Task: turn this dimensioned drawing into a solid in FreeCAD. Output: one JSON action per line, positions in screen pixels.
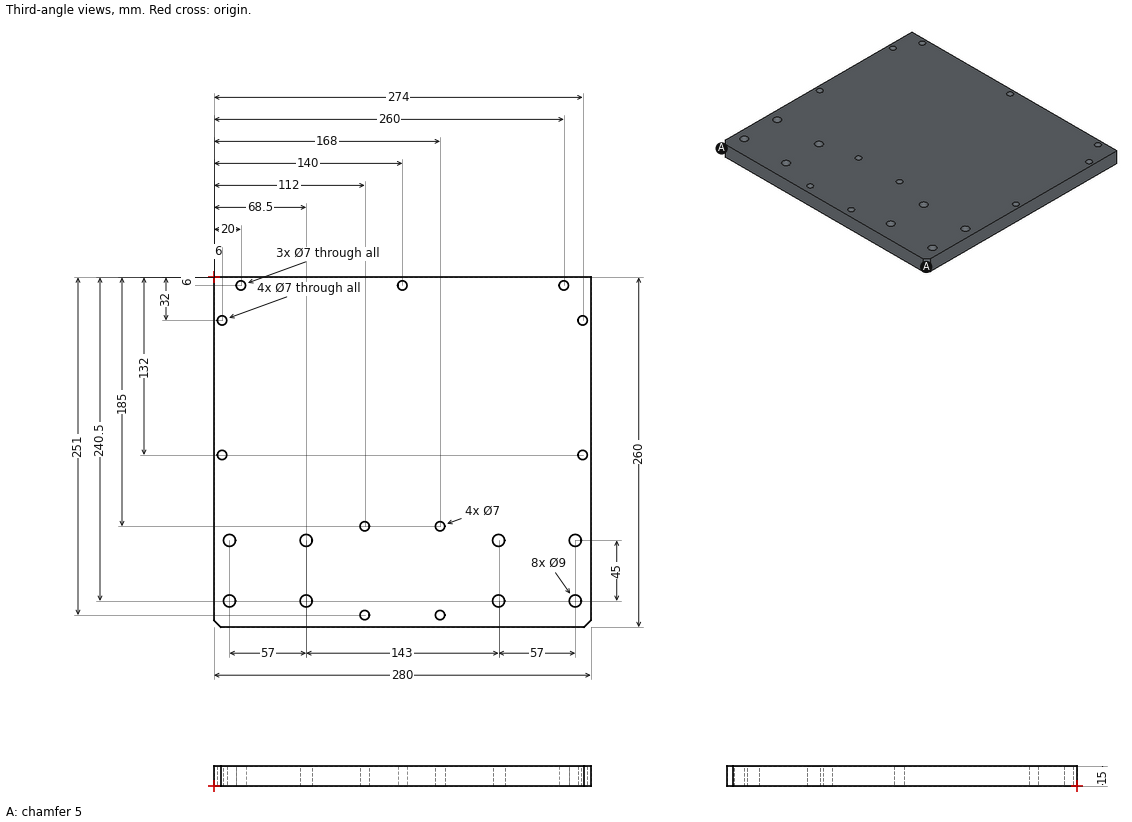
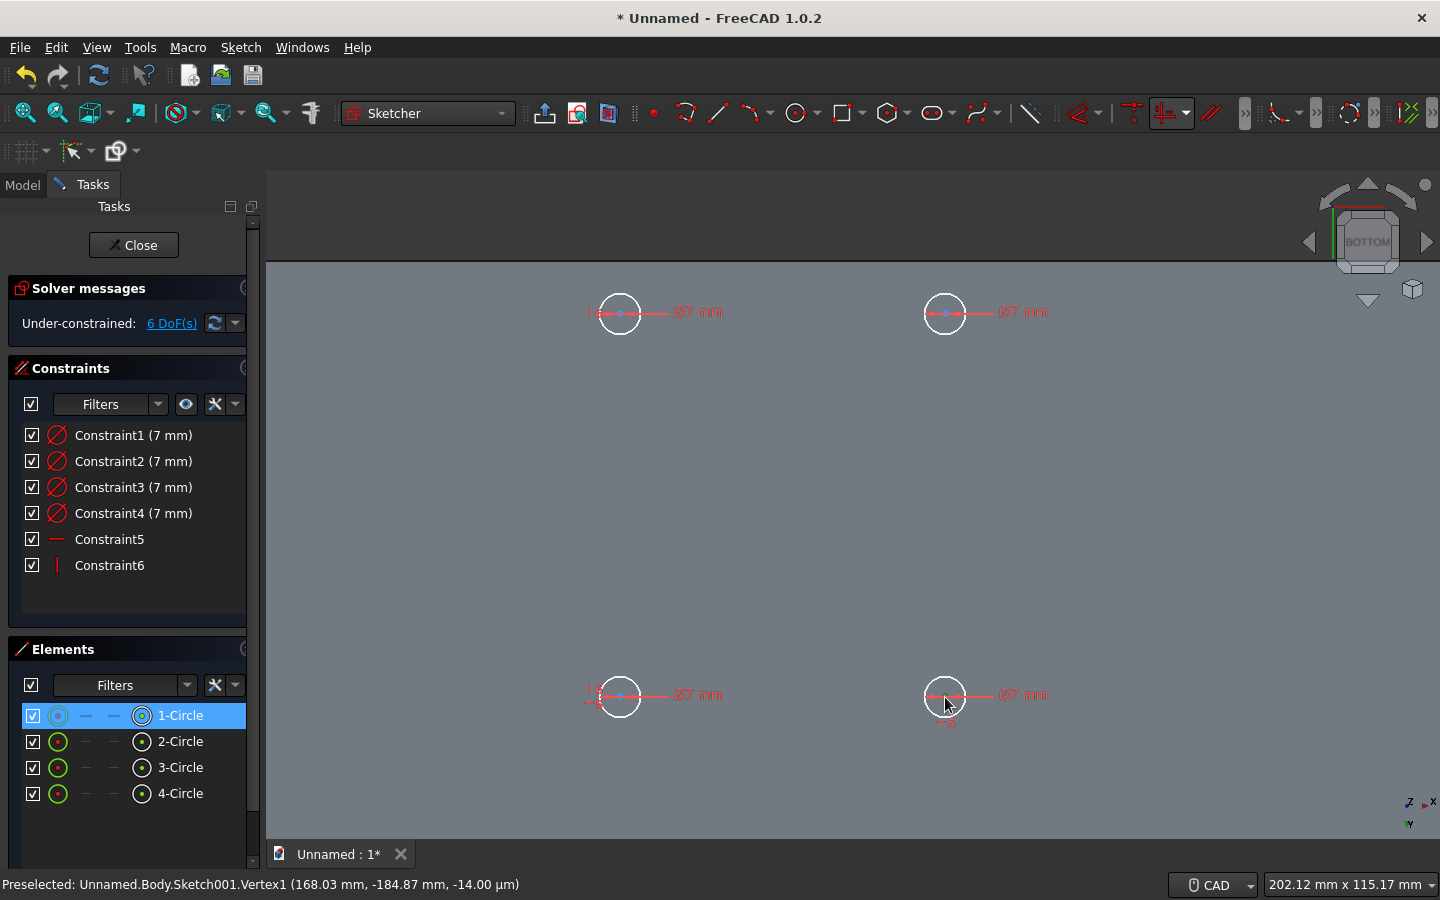
{"action": "left_click", "coordinate": [945, 314]}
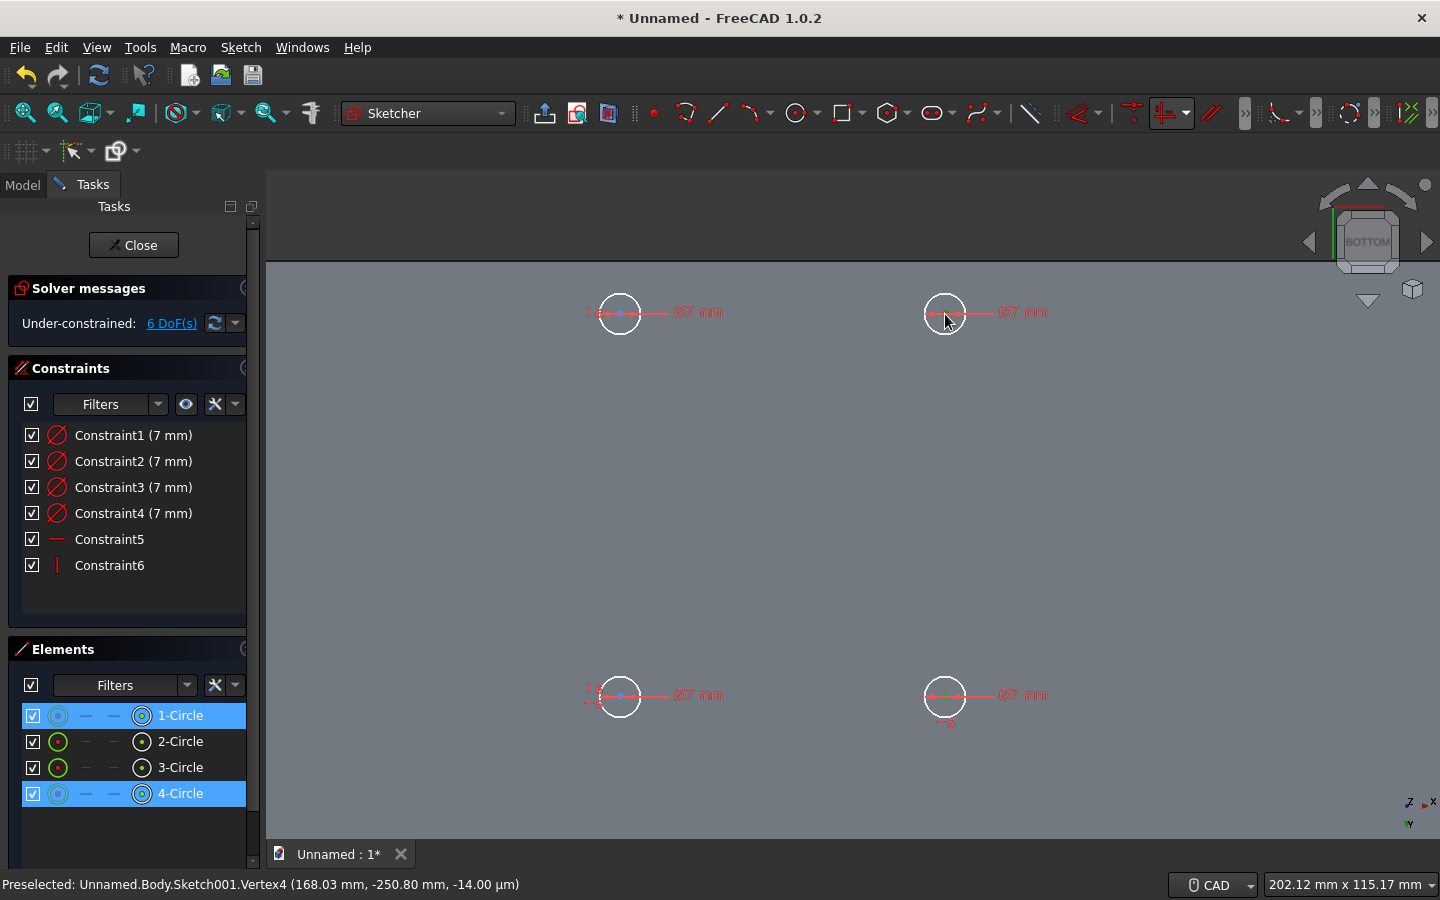
{"action": "left_click", "coordinate": [1188, 114]}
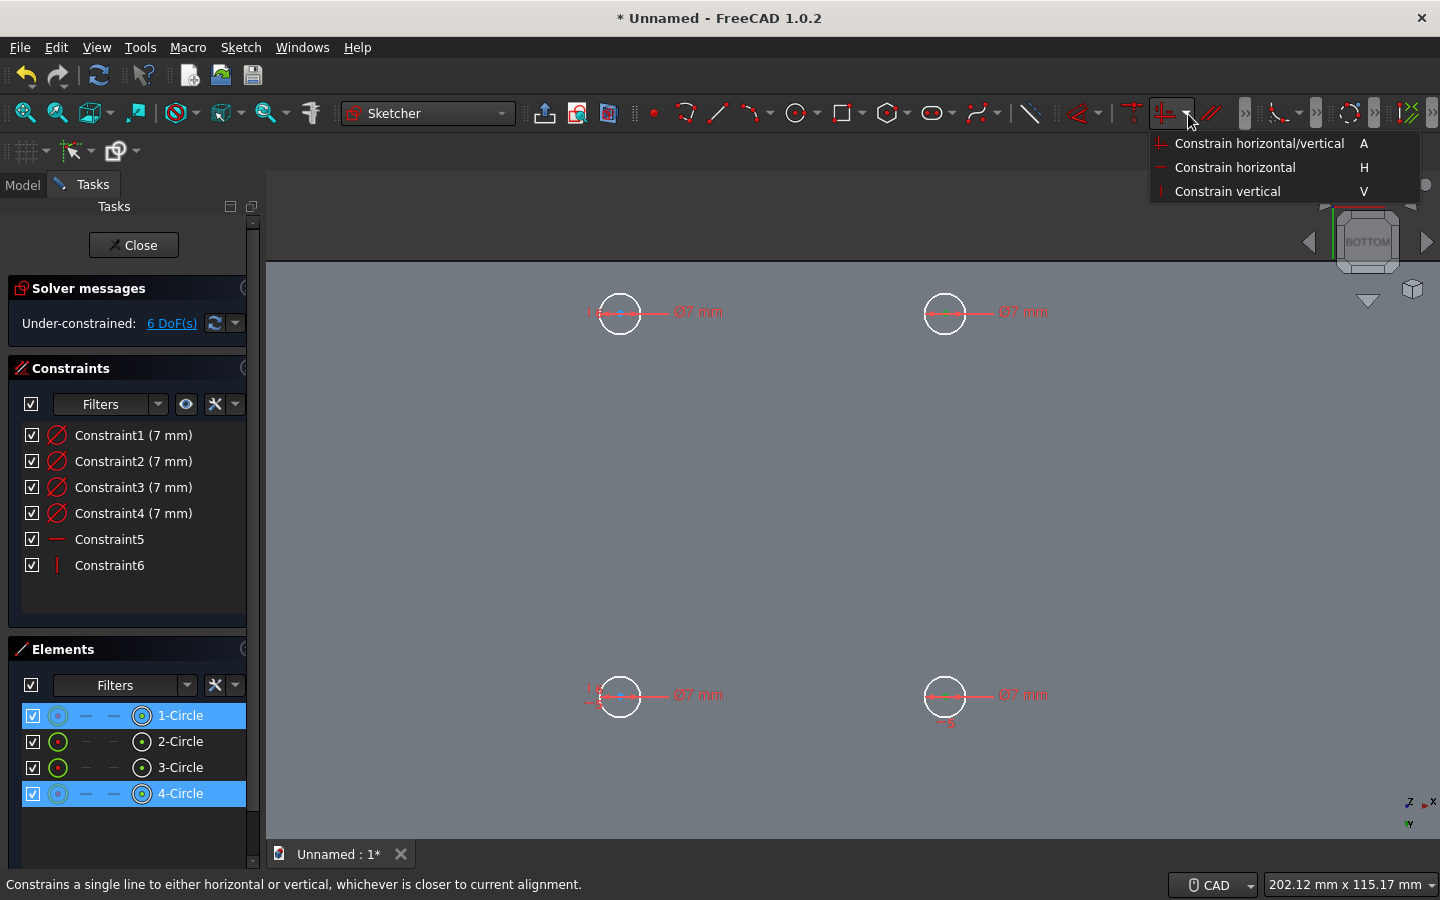
{"action": "left_click", "coordinate": [1285, 191]}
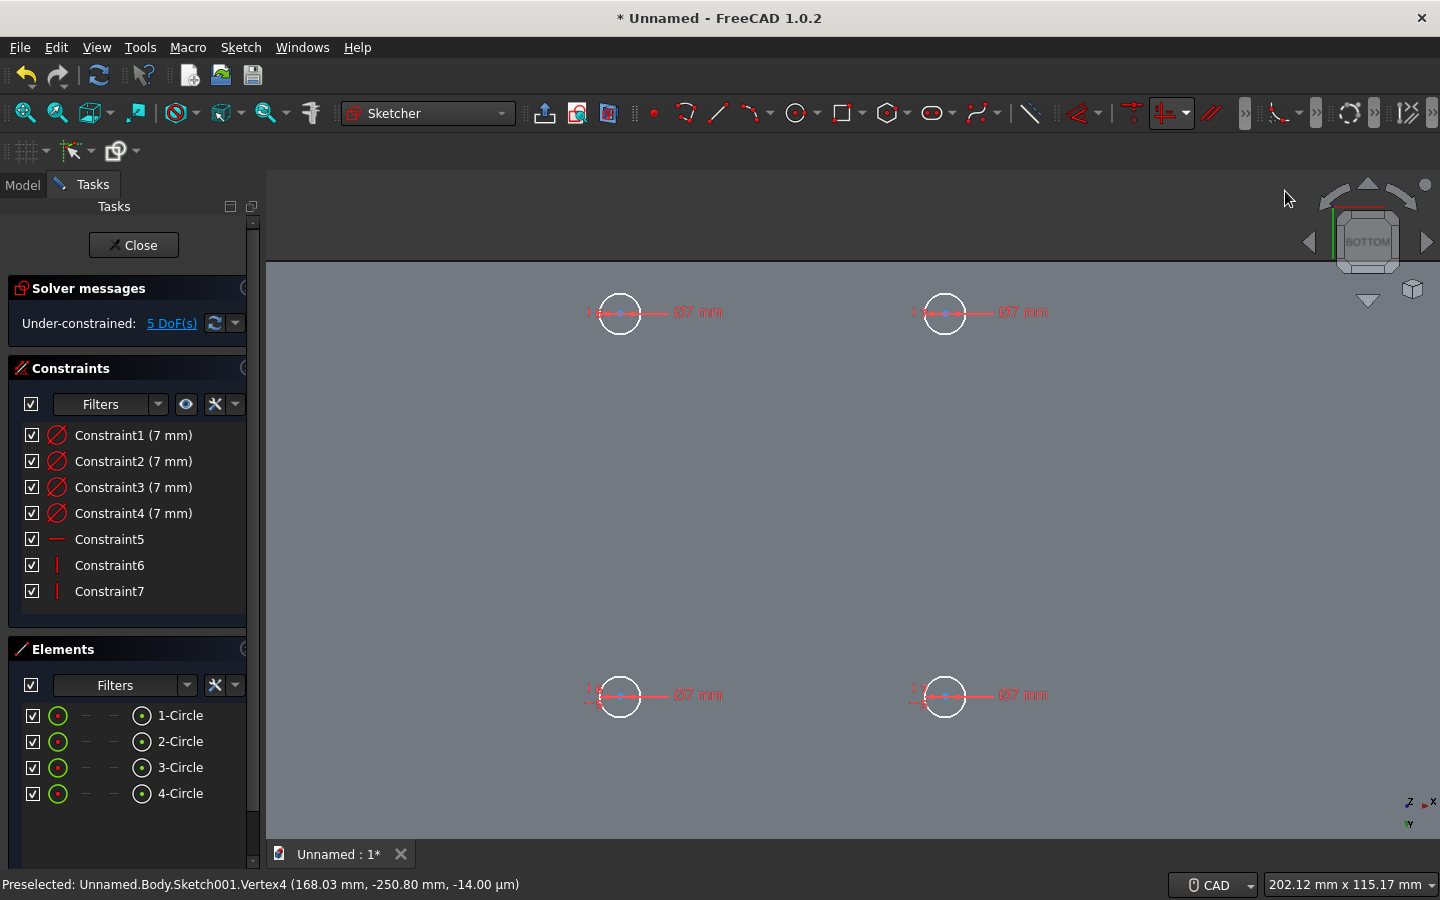
{"action": "left_click", "coordinate": [620, 314]}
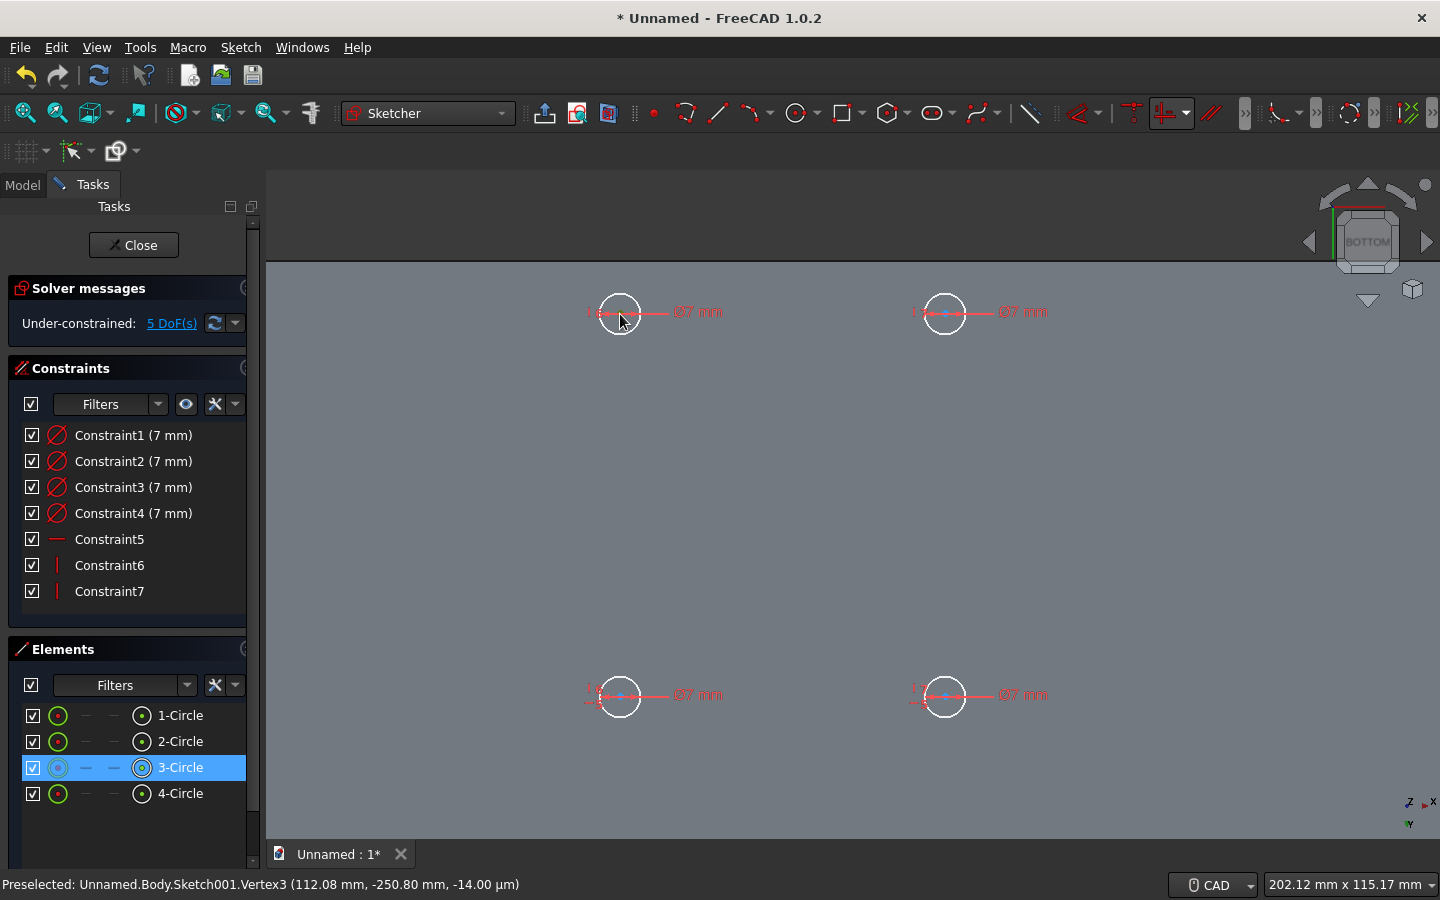
{"action": "left_click", "coordinate": [945, 314]}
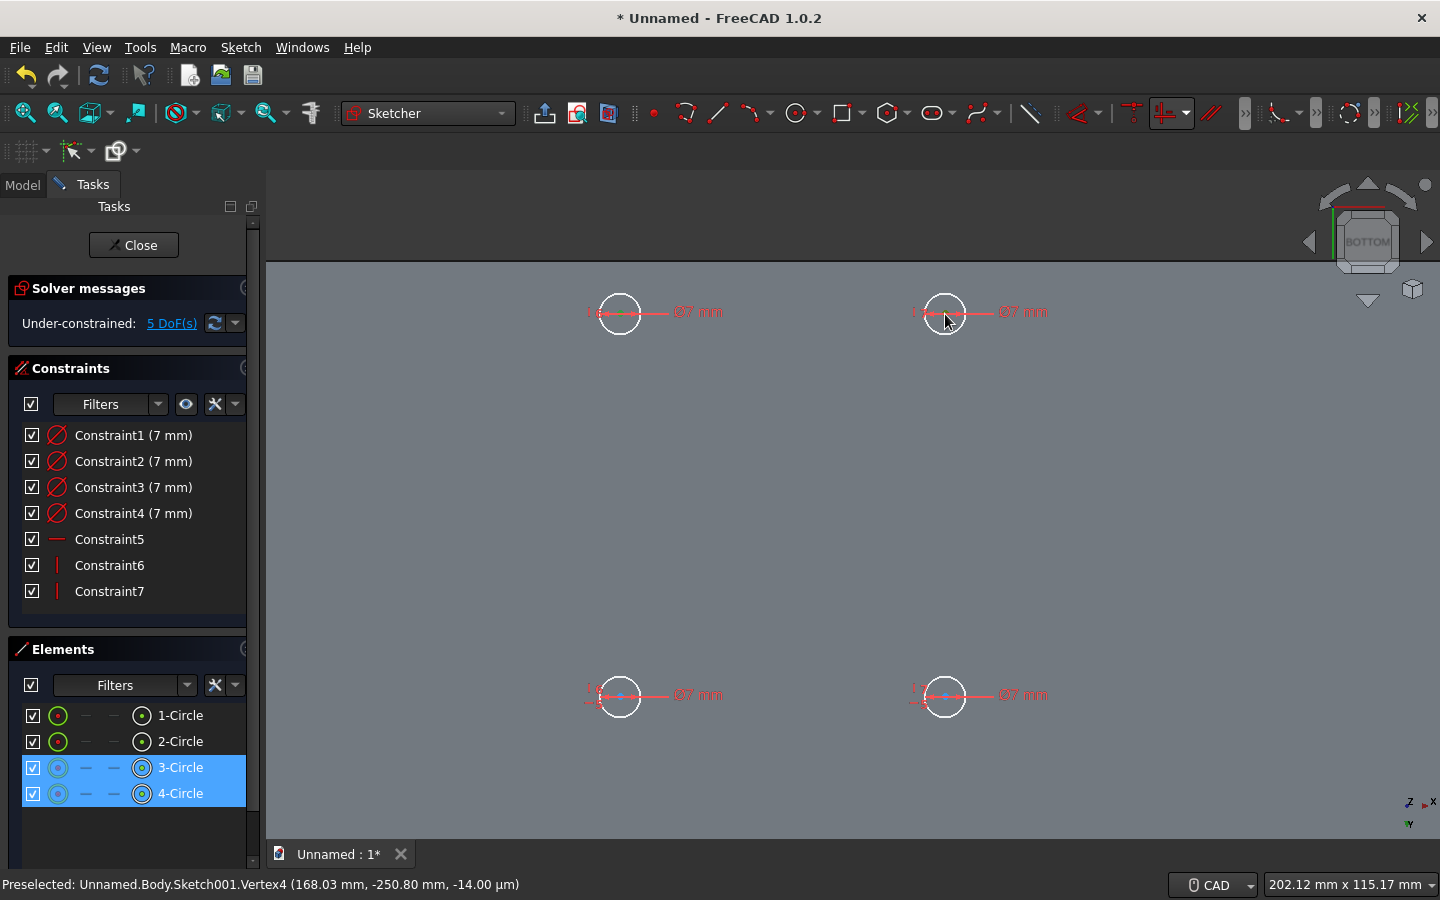
{"action": "key", "text": "h"}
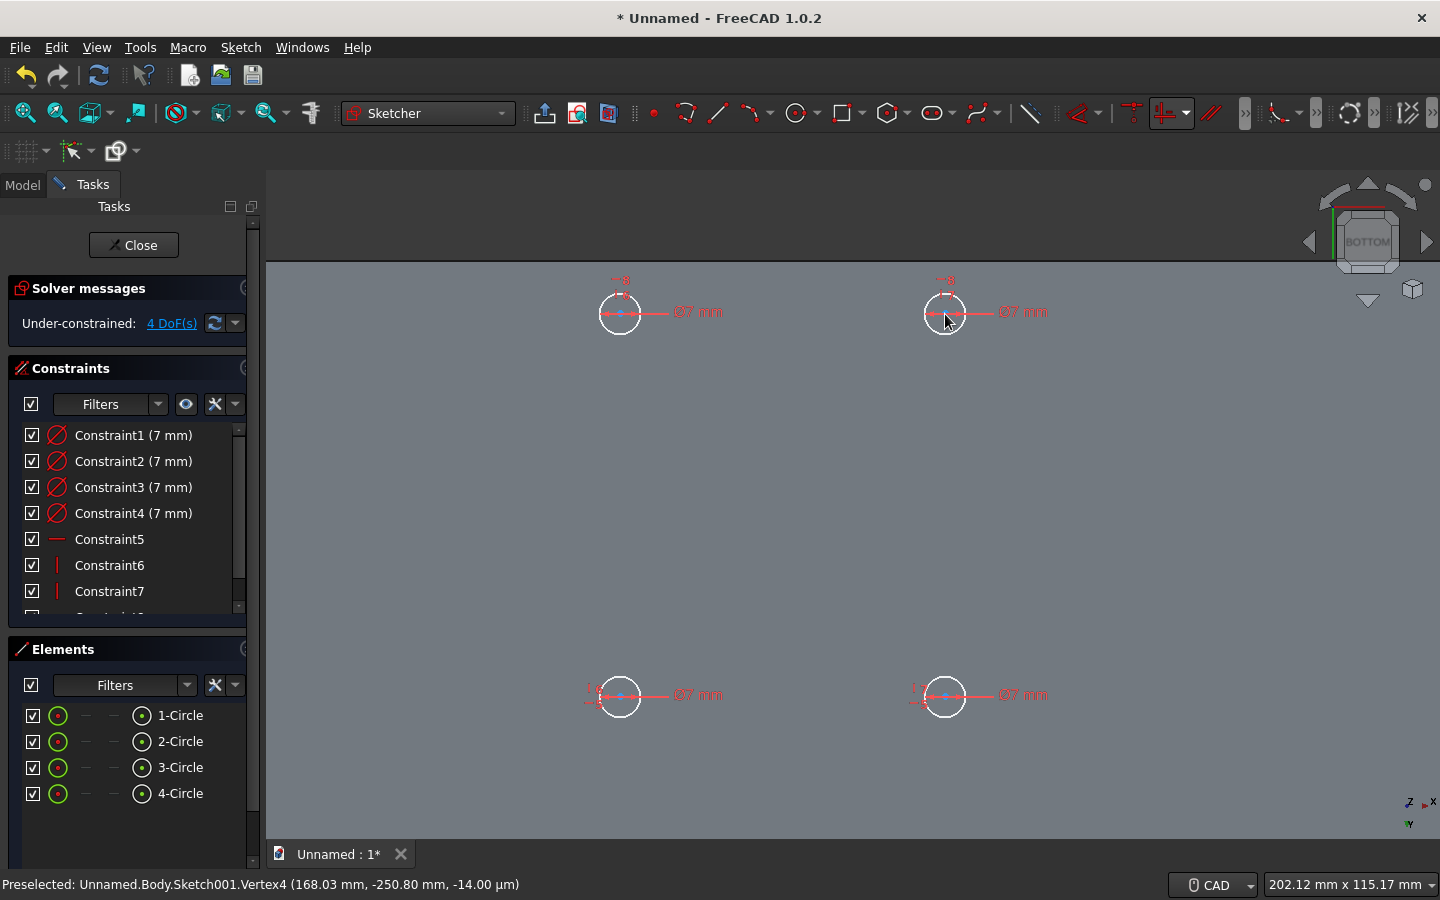
{"action": "left_click", "coordinate": [1078, 114]}